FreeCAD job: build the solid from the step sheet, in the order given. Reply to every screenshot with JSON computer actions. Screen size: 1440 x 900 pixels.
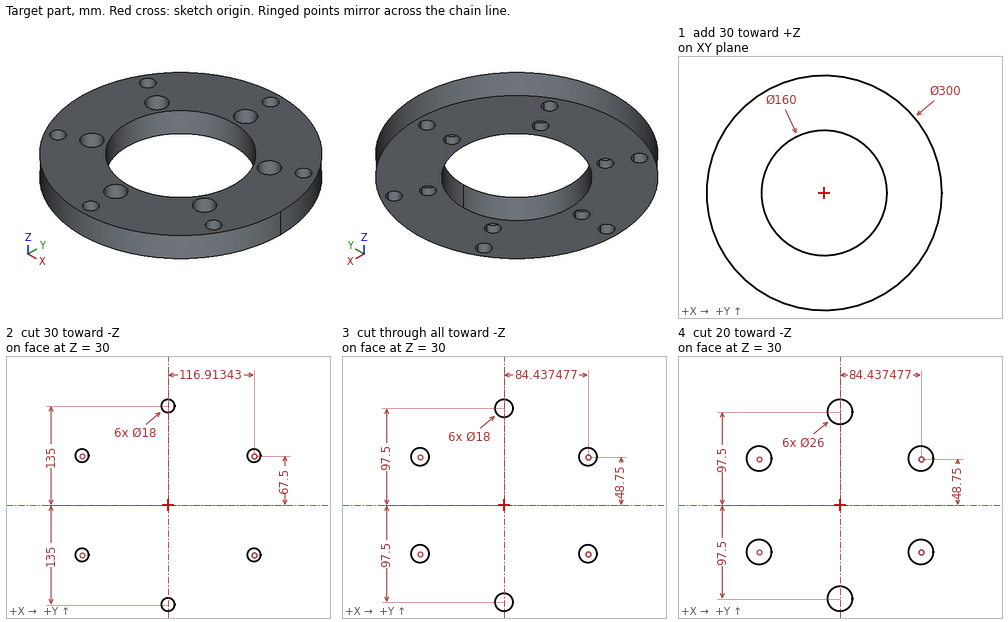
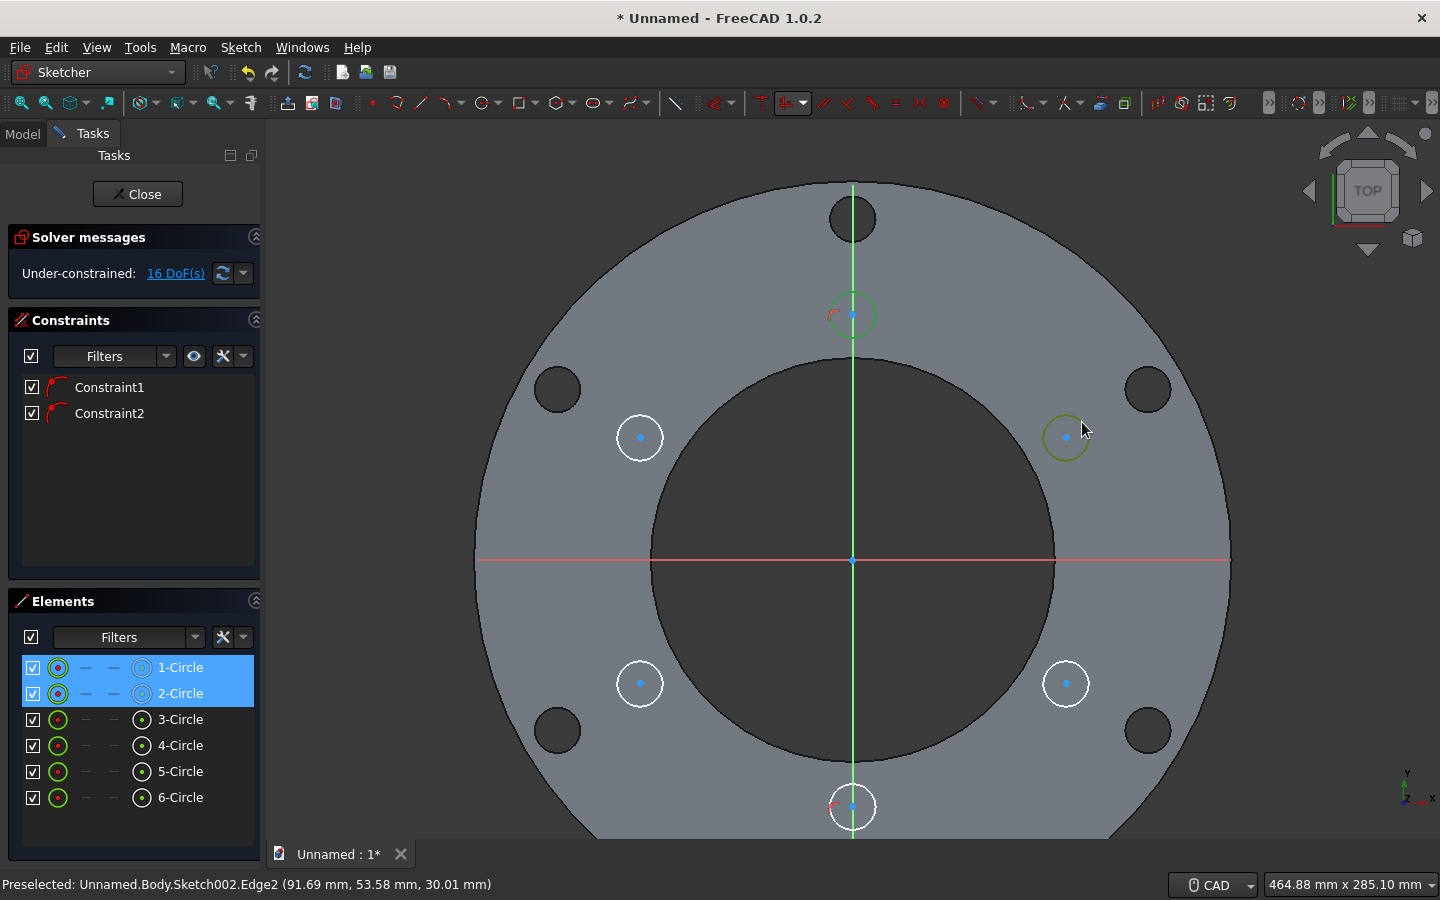
{"action": "left_click", "coordinate": [1082, 668]}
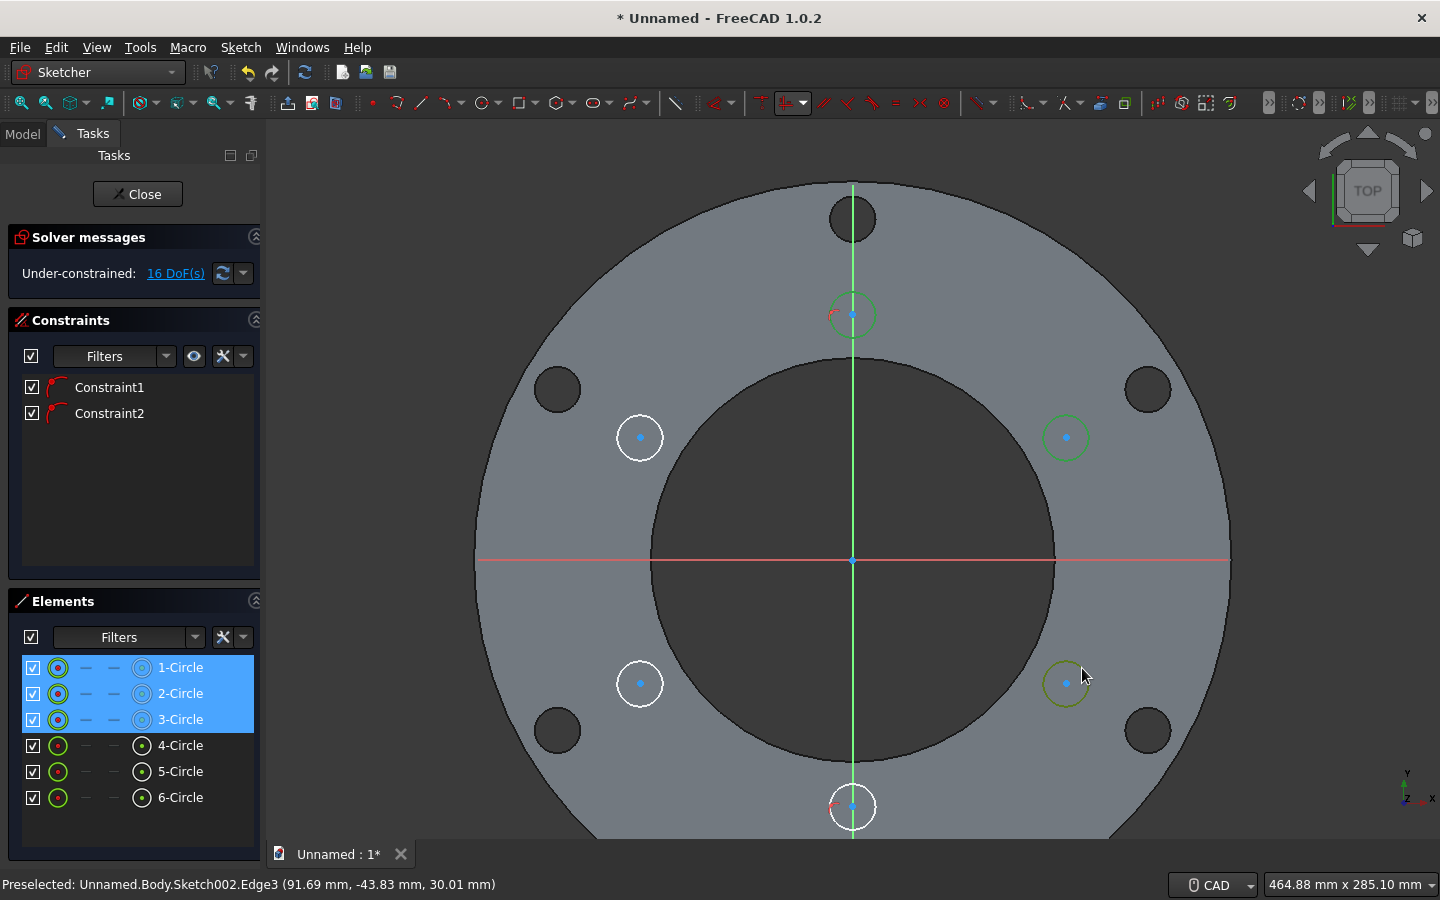
{"action": "left_click", "coordinate": [869, 791]}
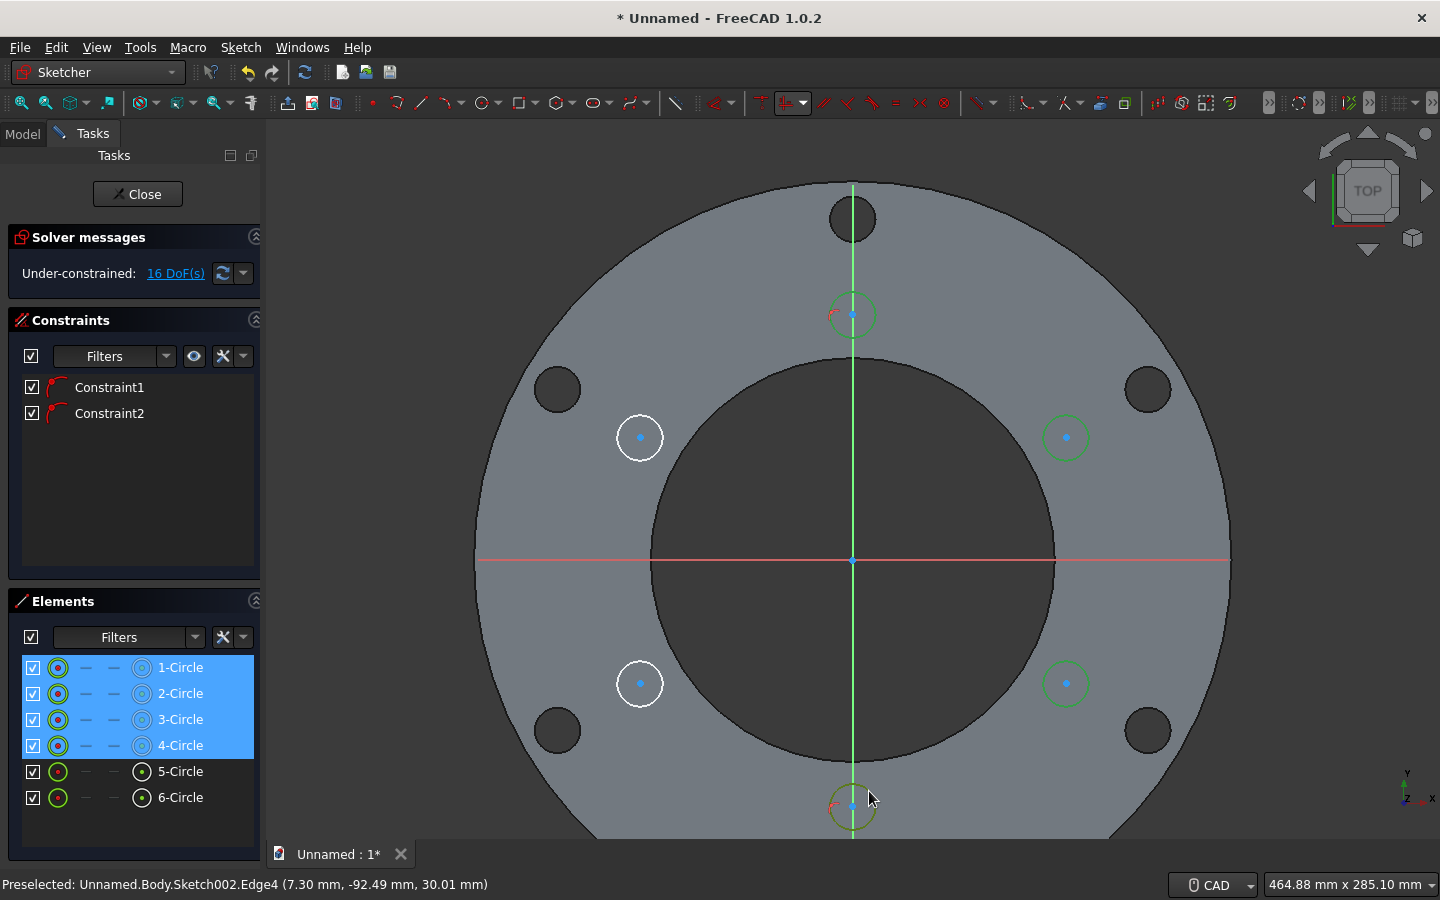
{"action": "left_click", "coordinate": [656, 668]}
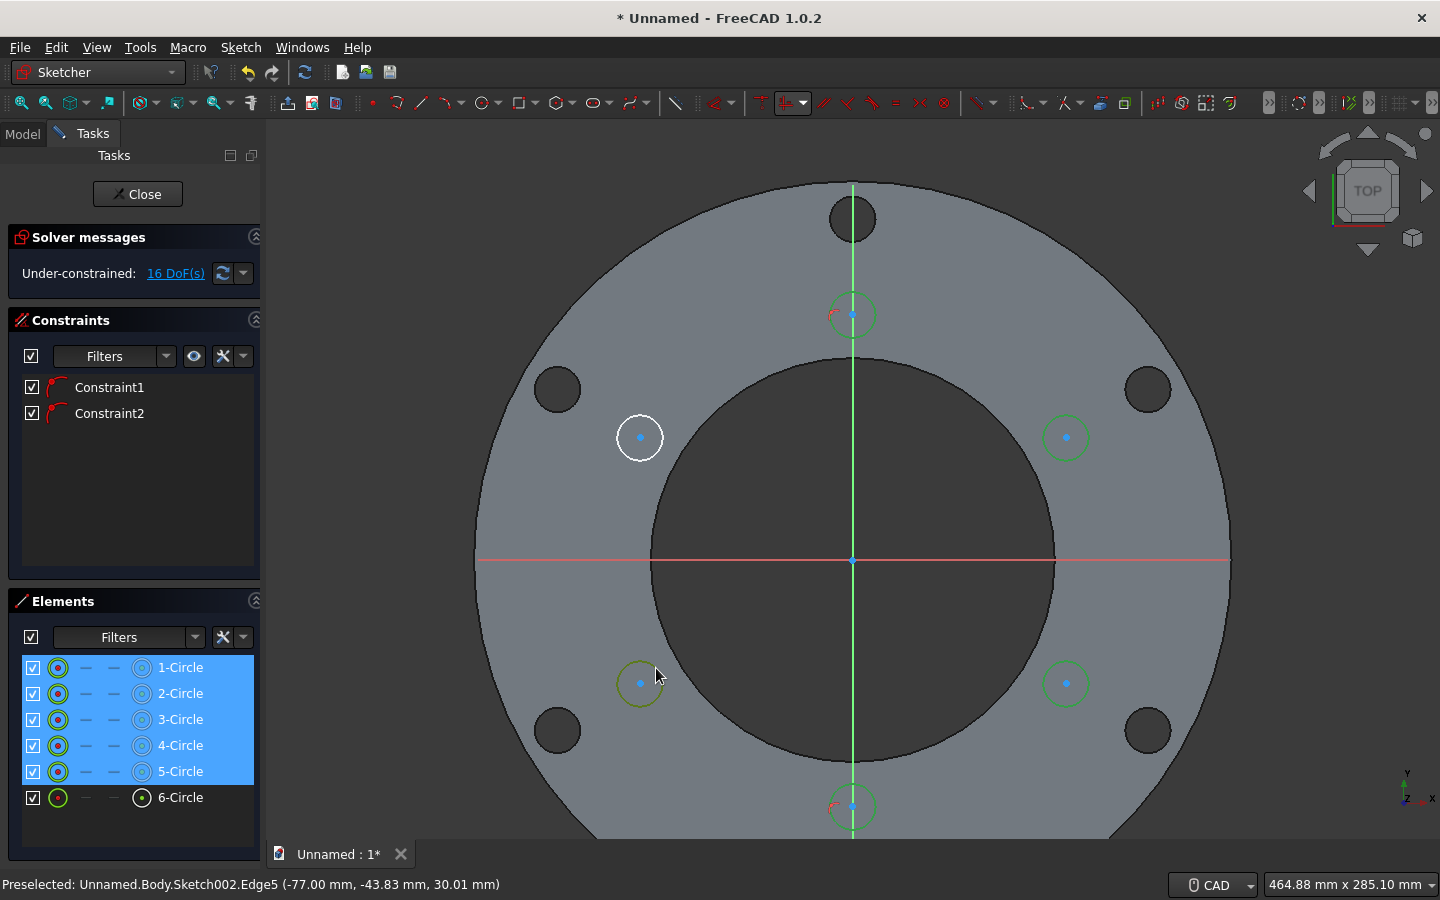
{"action": "left_click", "coordinate": [656, 422]}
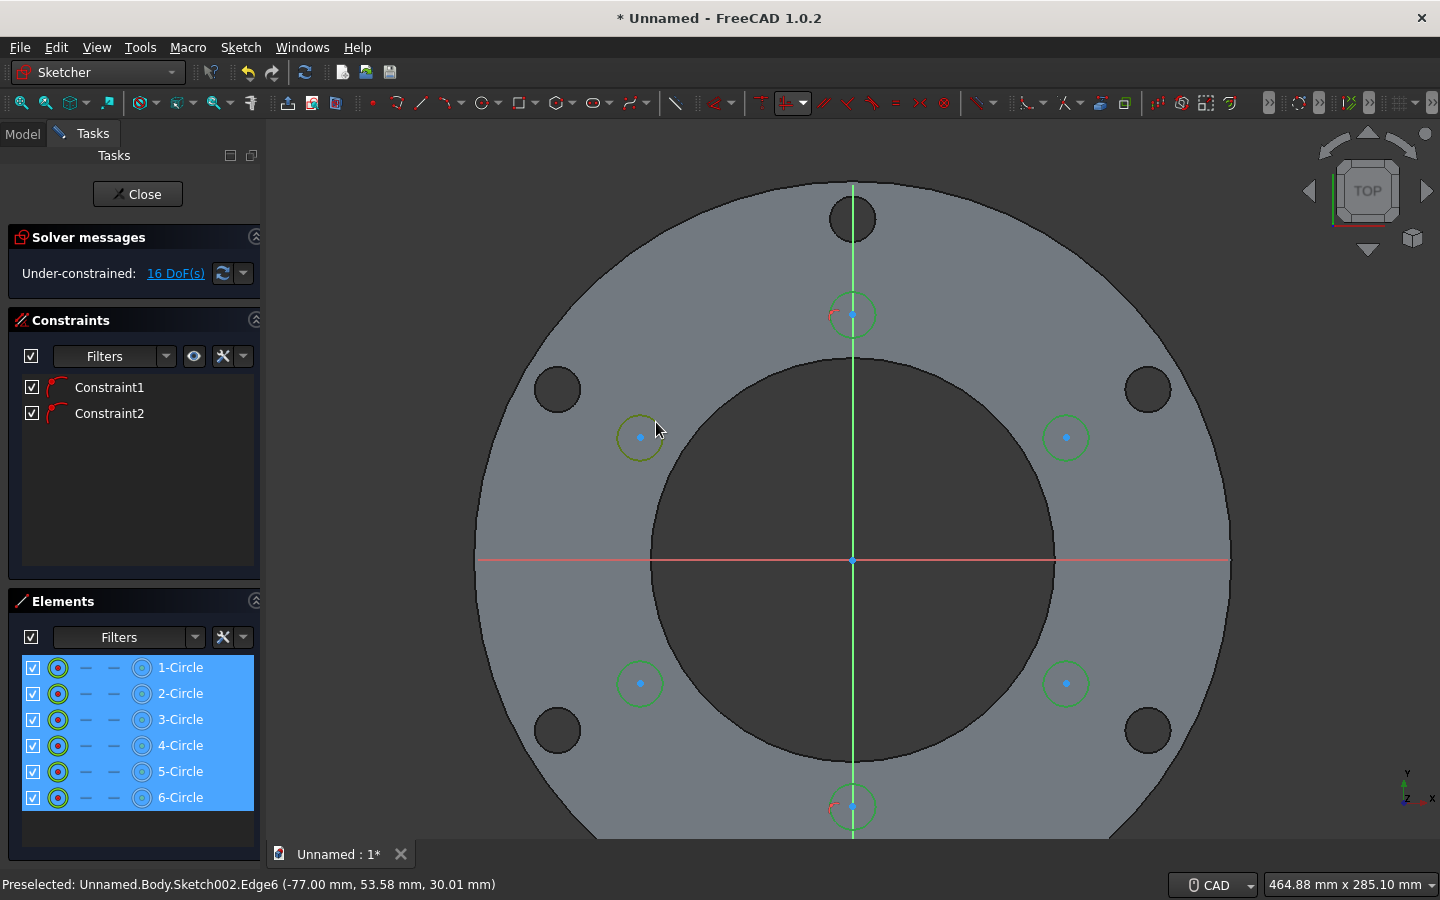
{"action": "key", "text": "e"}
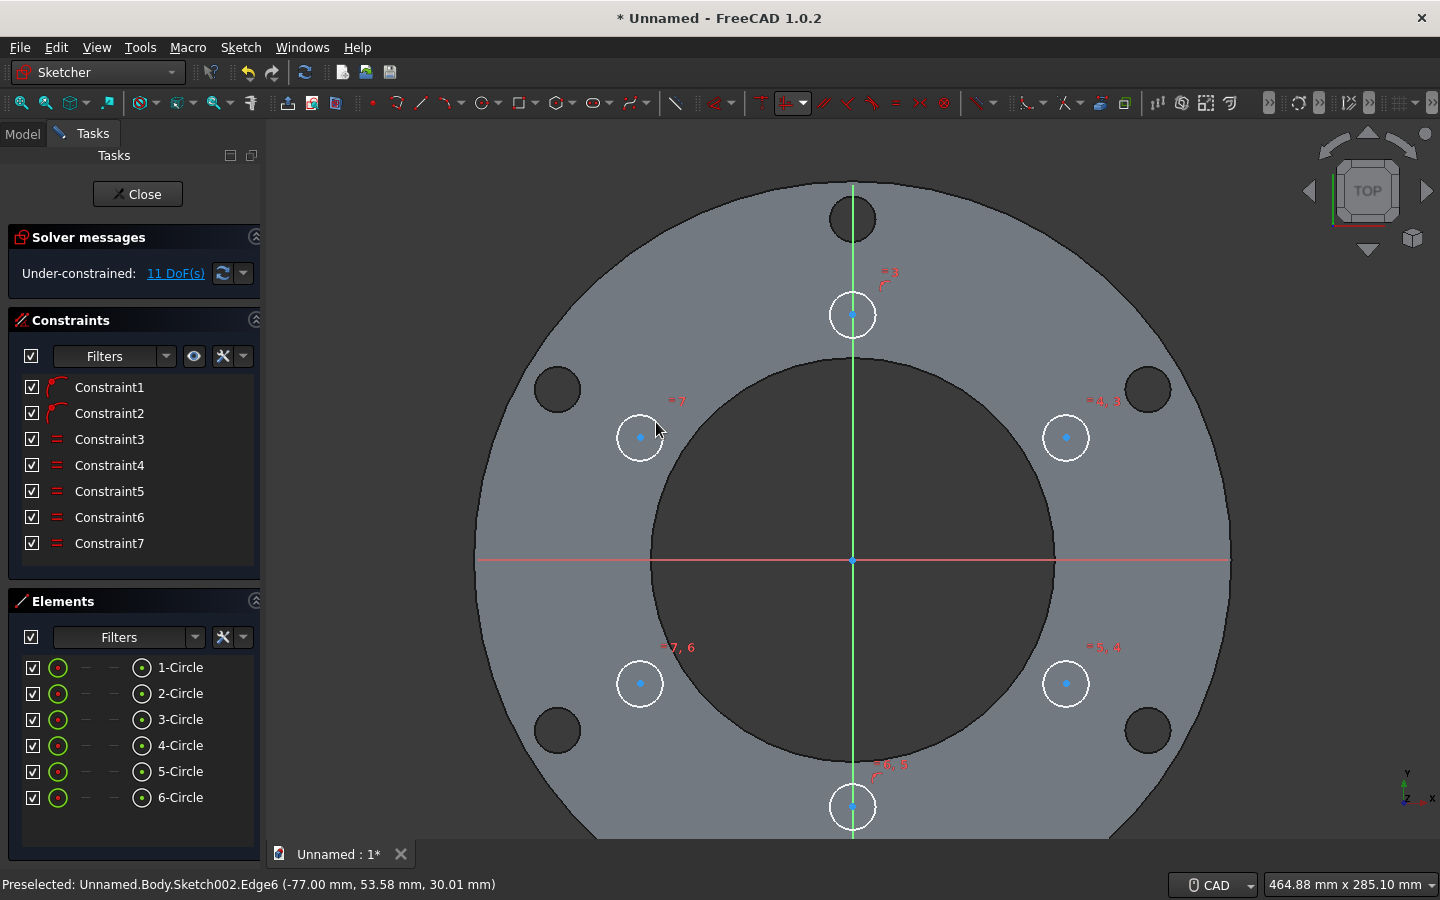
{"action": "left_click", "coordinate": [1066, 438]}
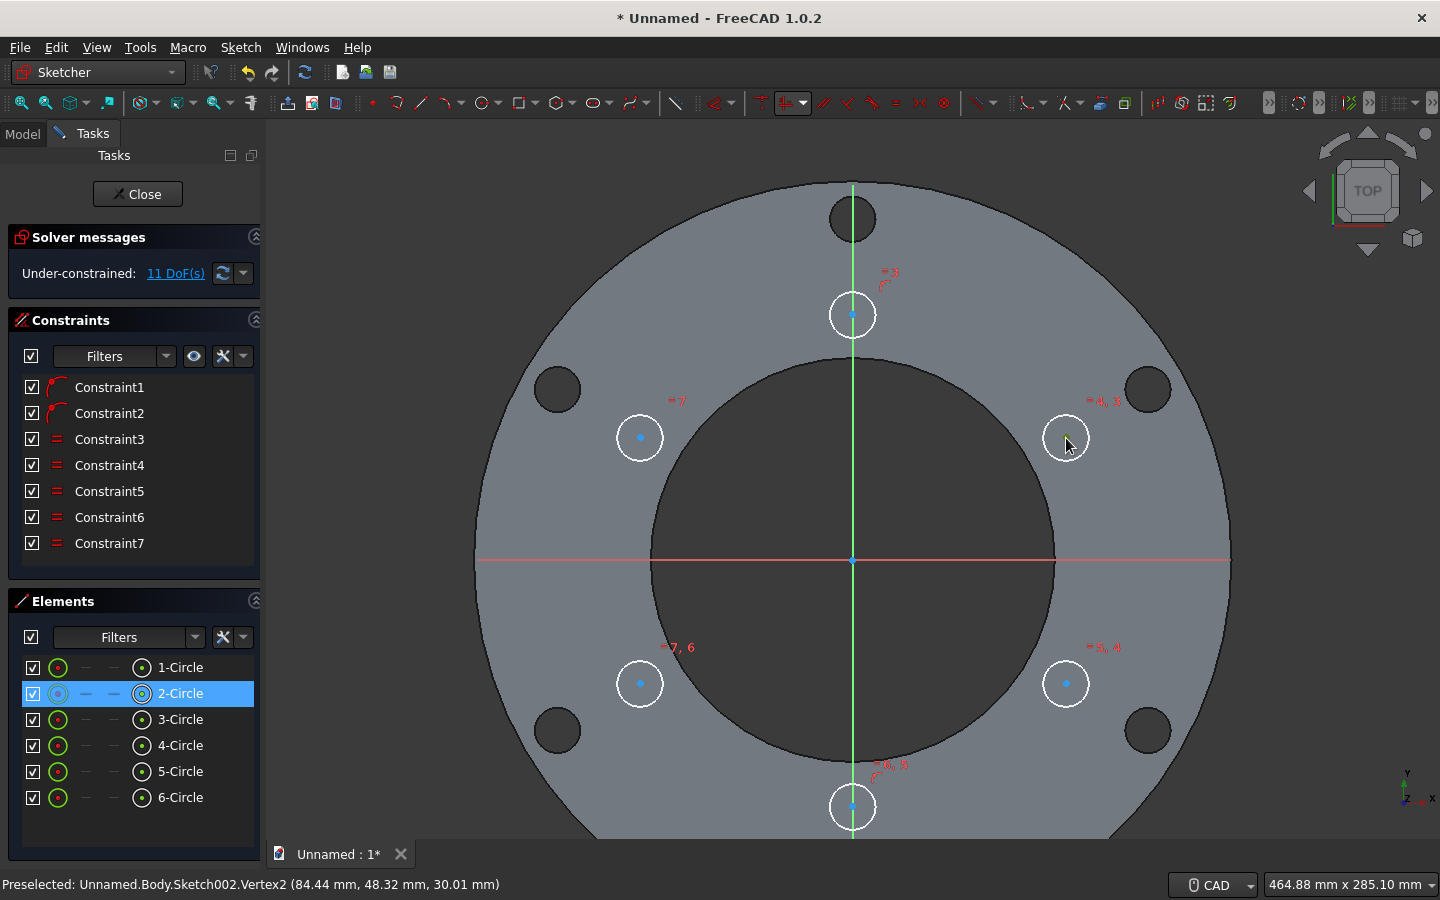
{"action": "left_click", "coordinate": [1066, 684]}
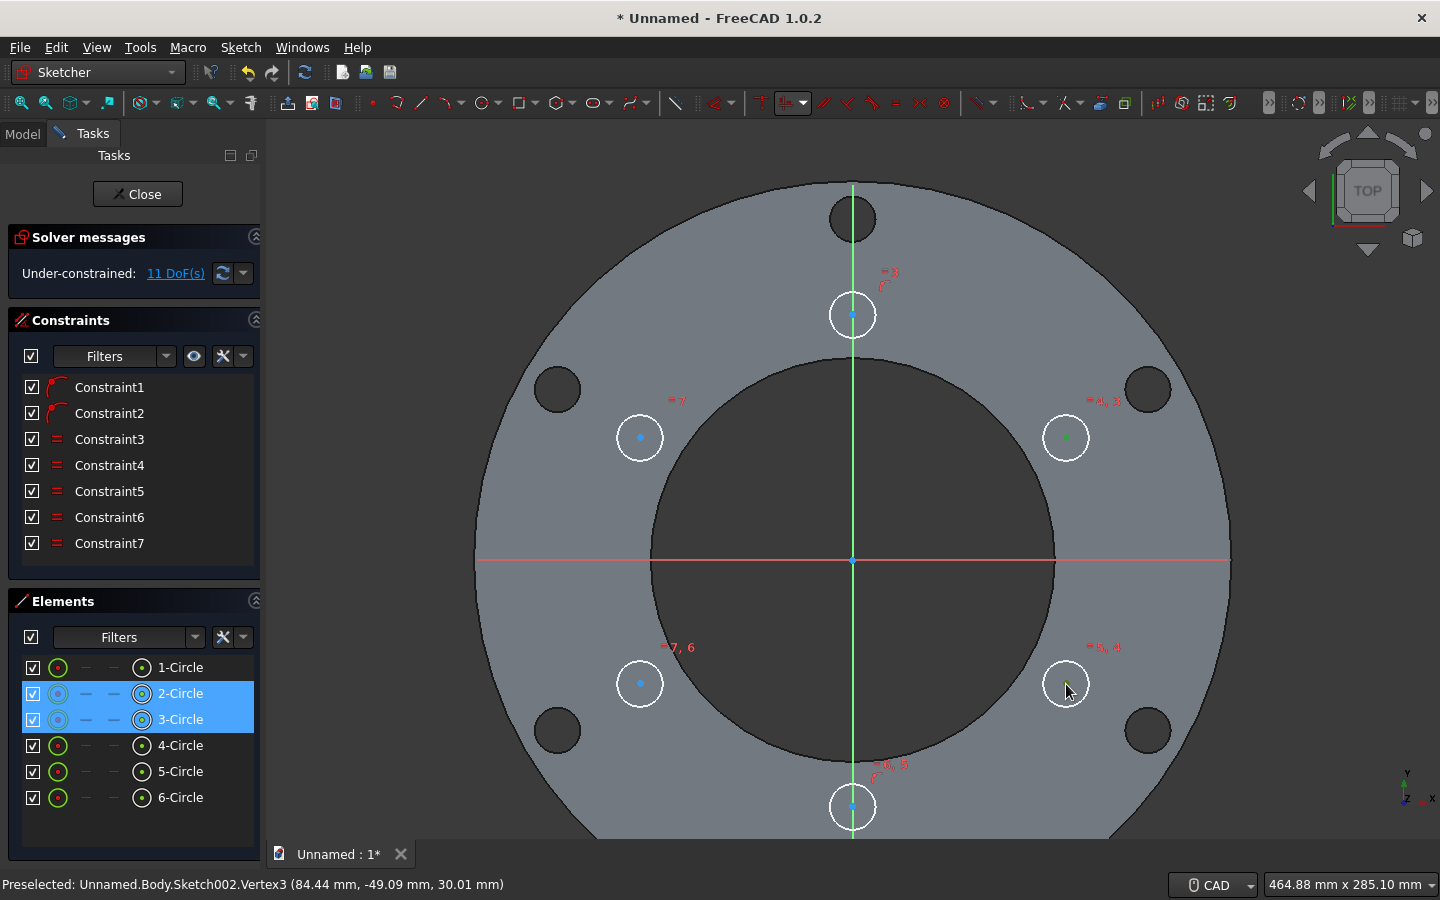
{"action": "left_click", "coordinate": [504, 560]}